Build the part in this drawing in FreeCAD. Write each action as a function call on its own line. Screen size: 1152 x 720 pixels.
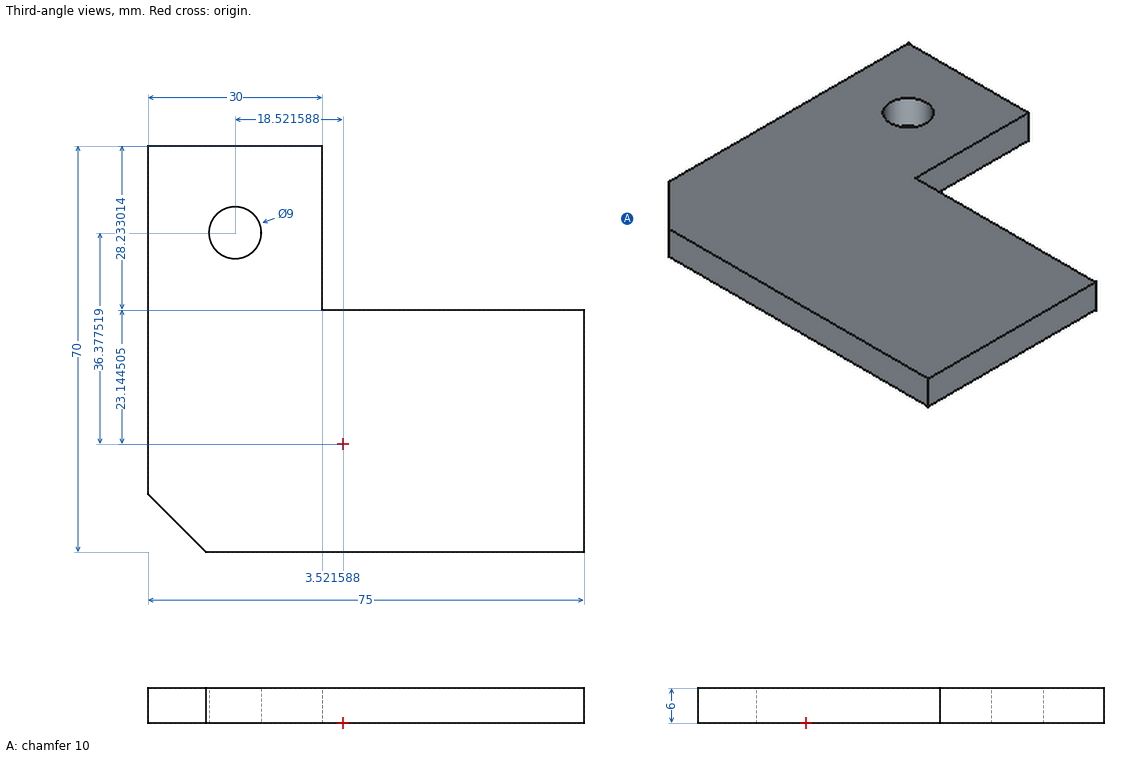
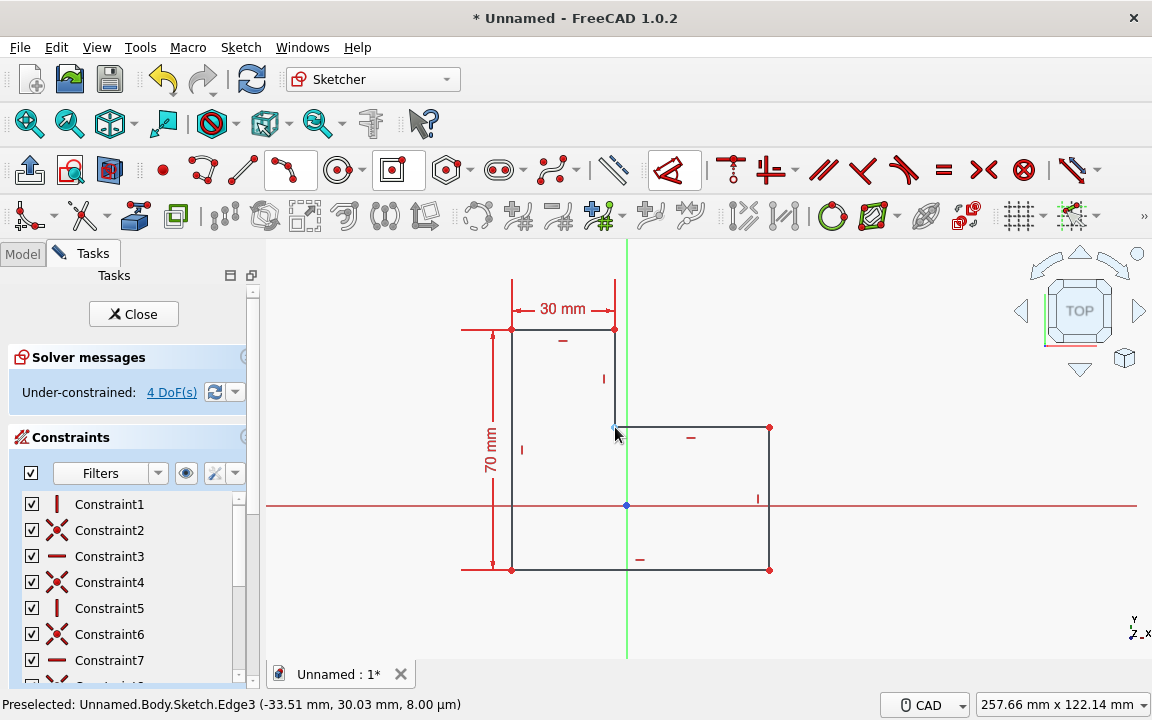
click(589, 570)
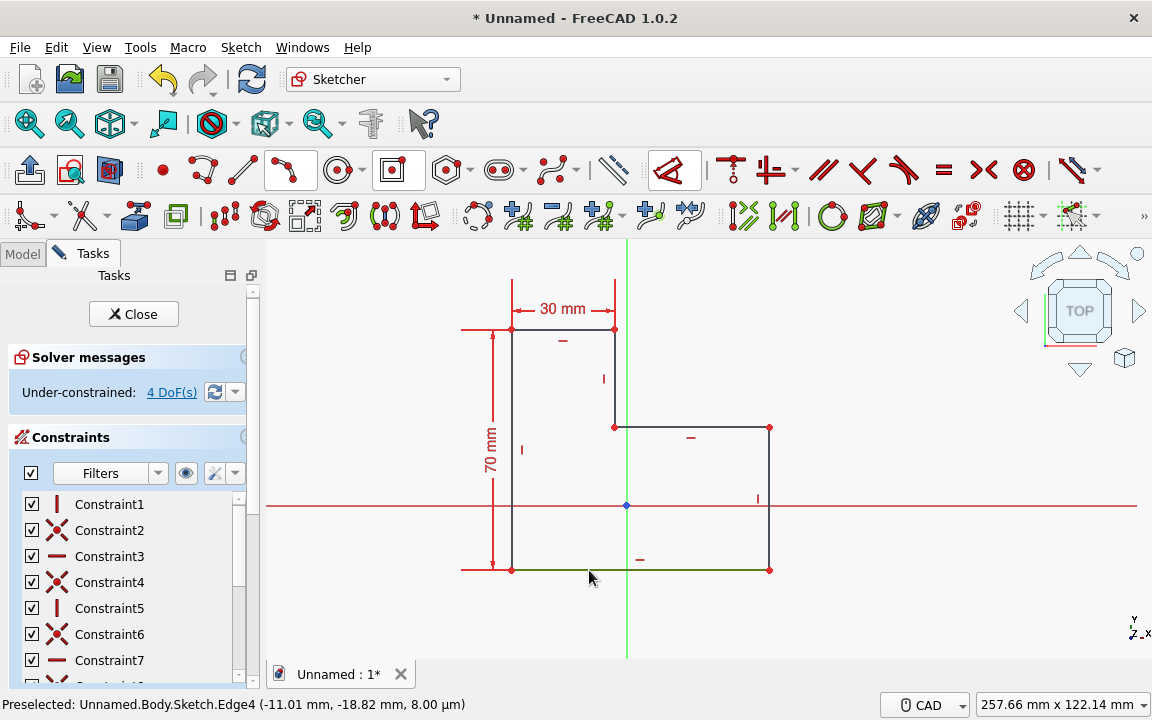
key(l)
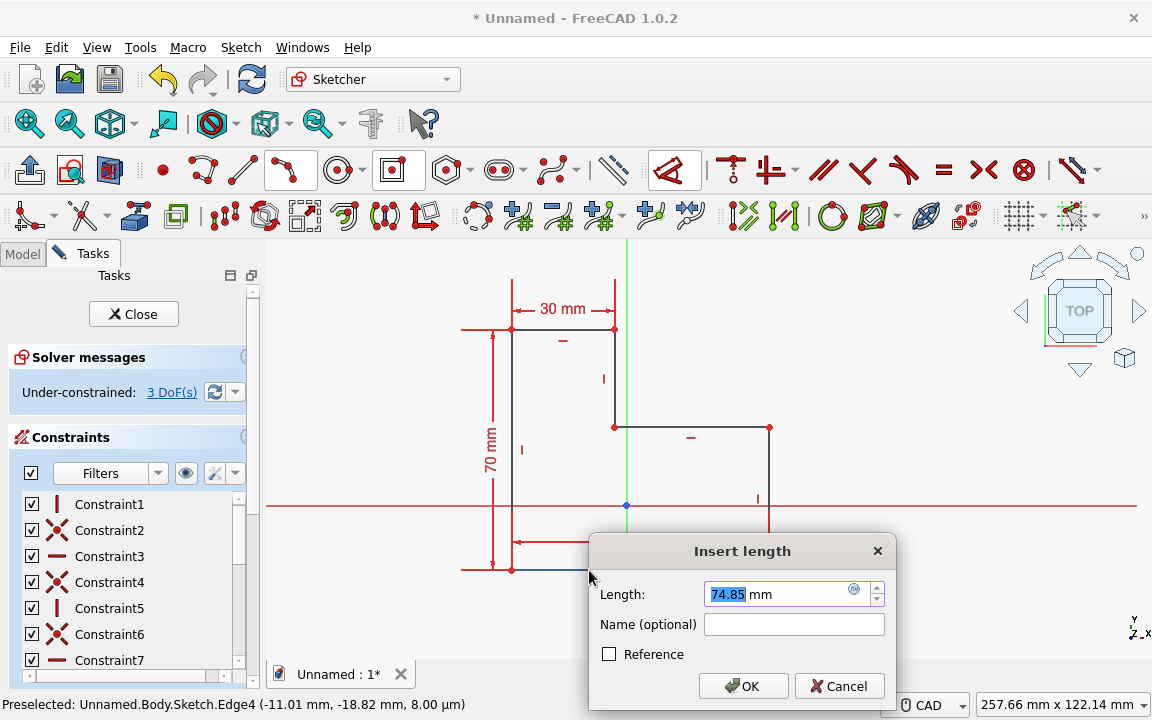
text(75)
key(Return)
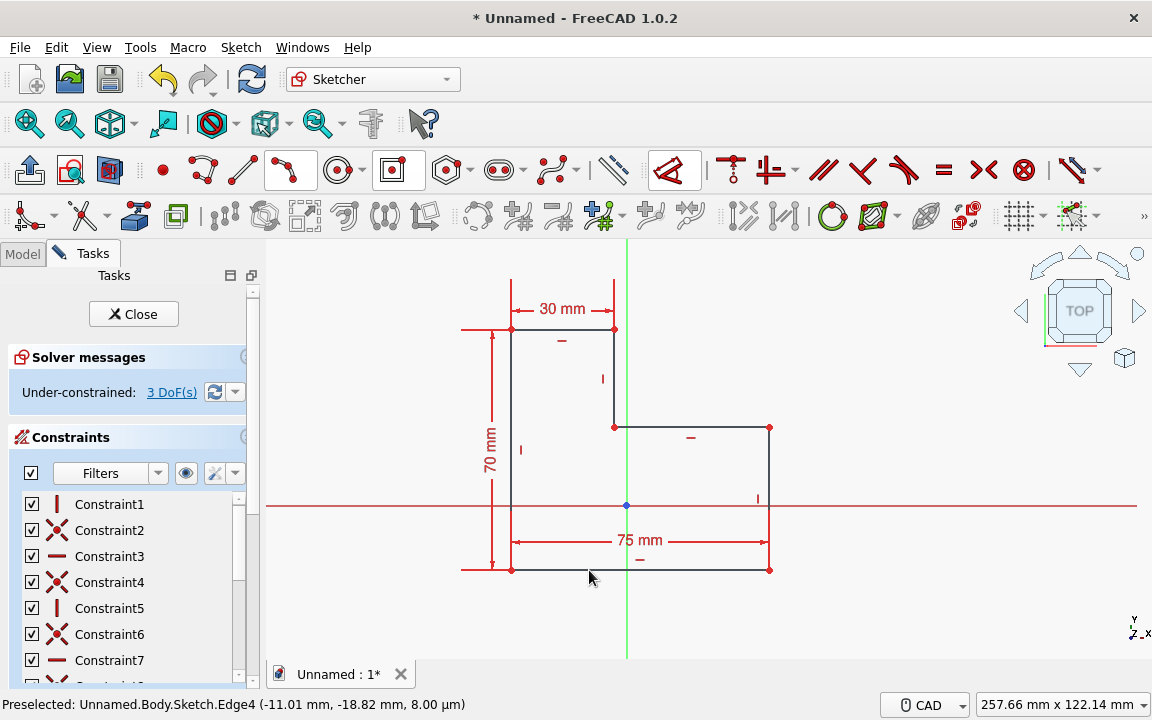
click(614, 398)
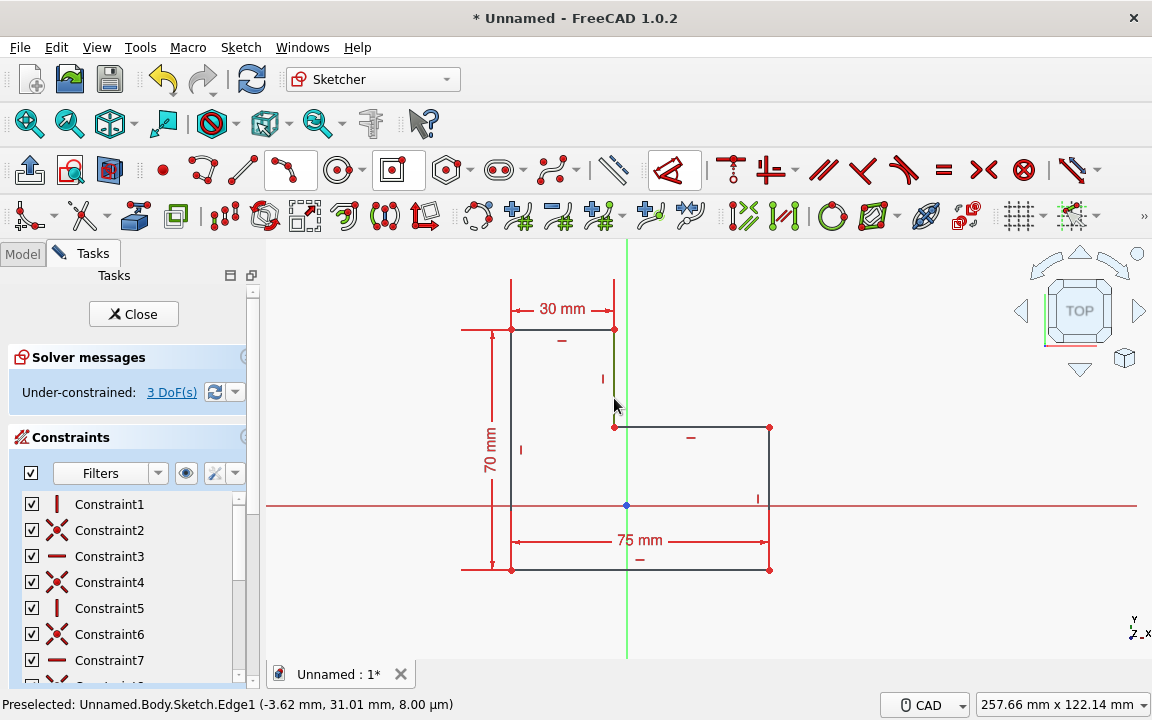
click(696, 170)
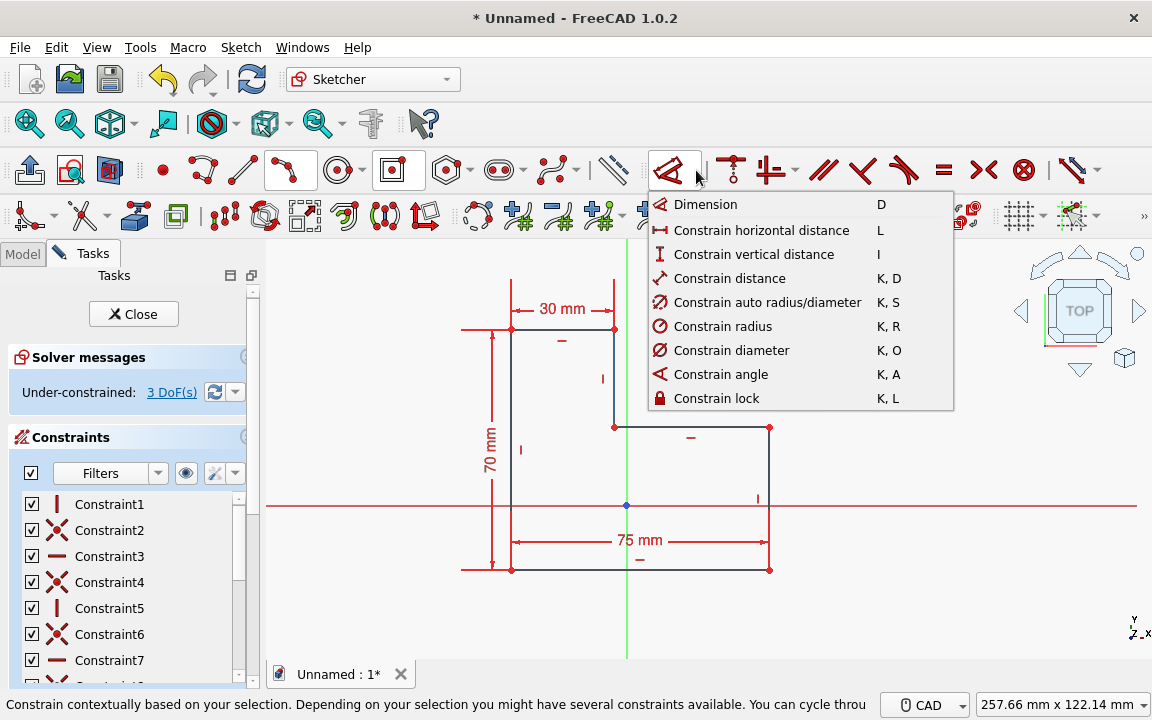
click(801, 254)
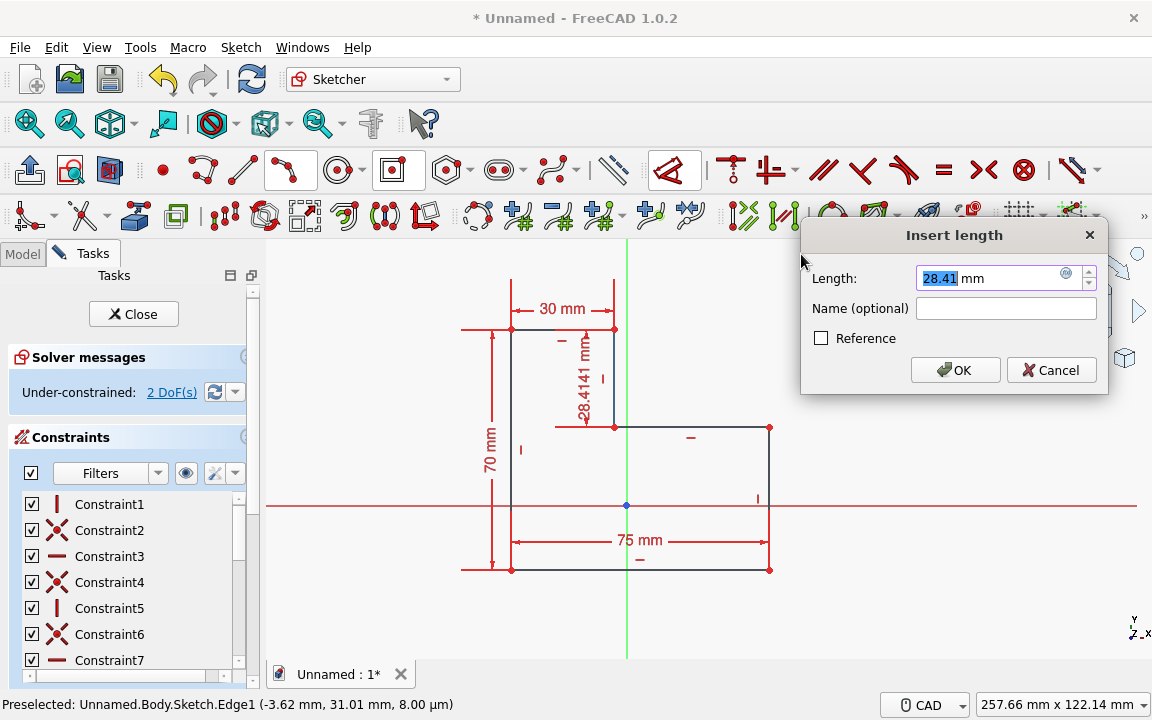
text(28.233014)
key(Return)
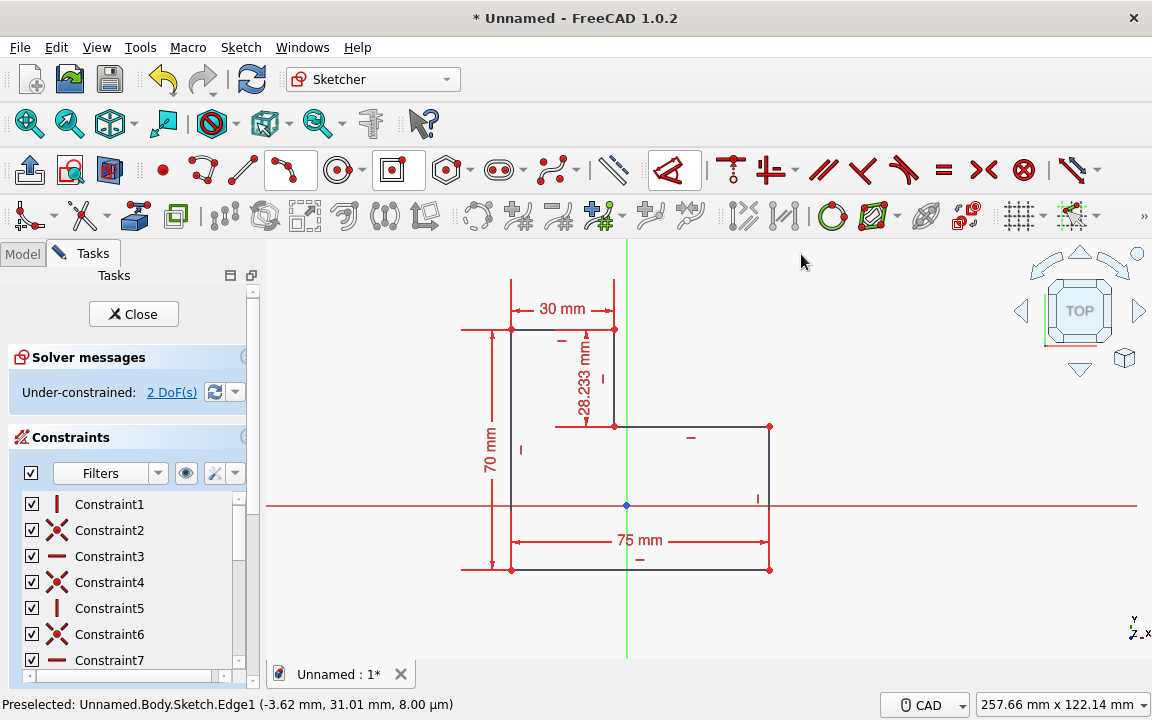
scroll(614, 427, up, 6)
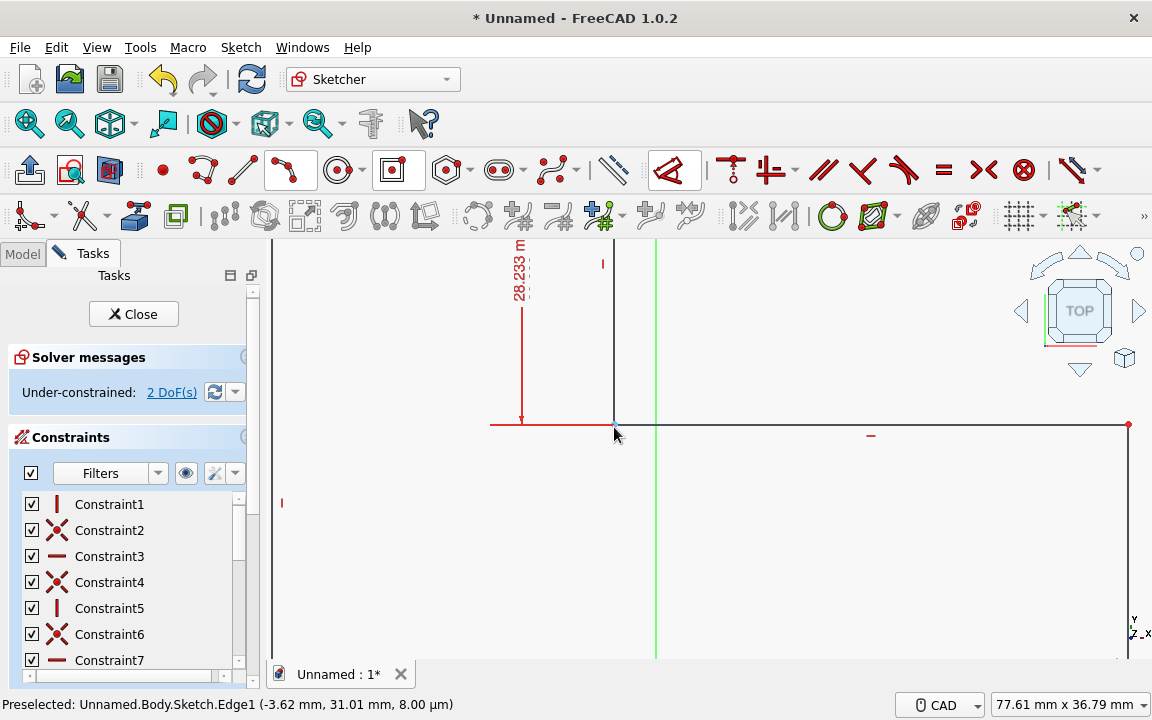
click(614, 425)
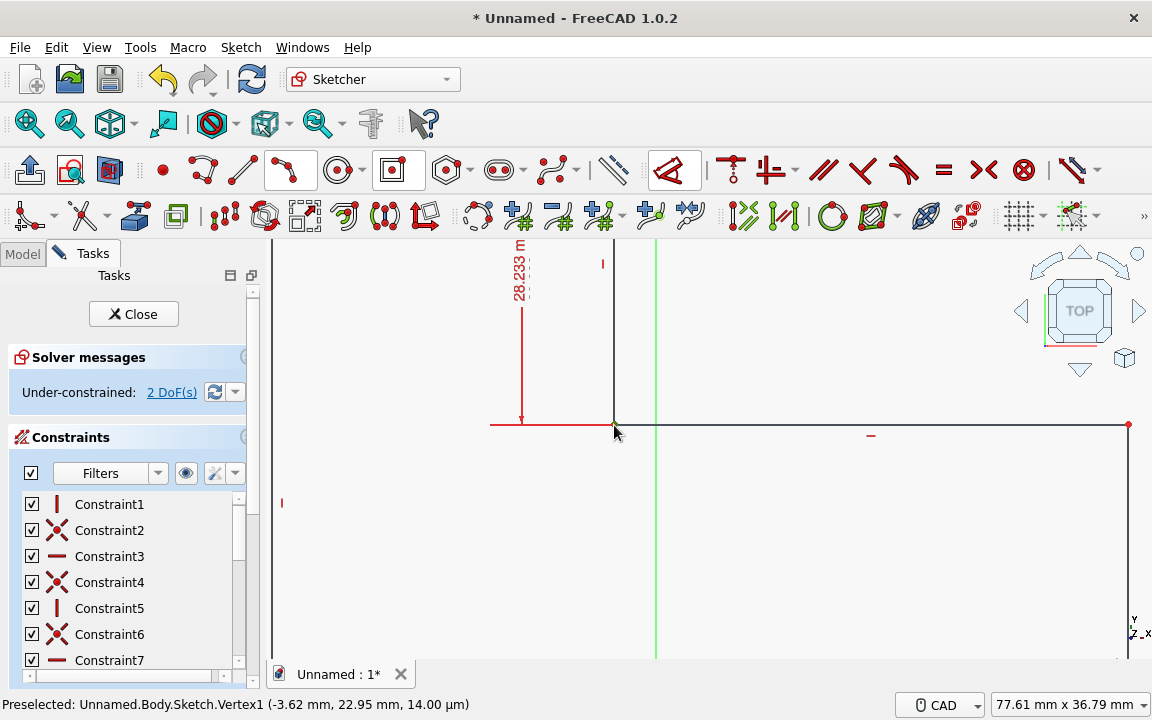
click(696, 170)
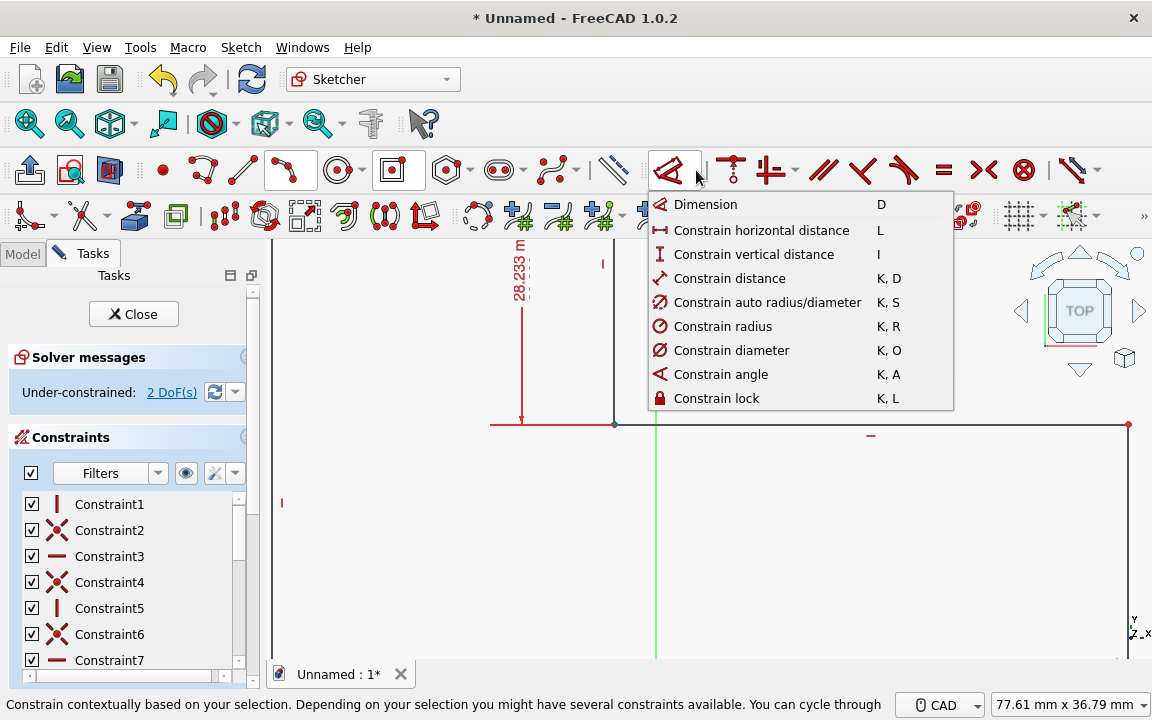
click(801, 230)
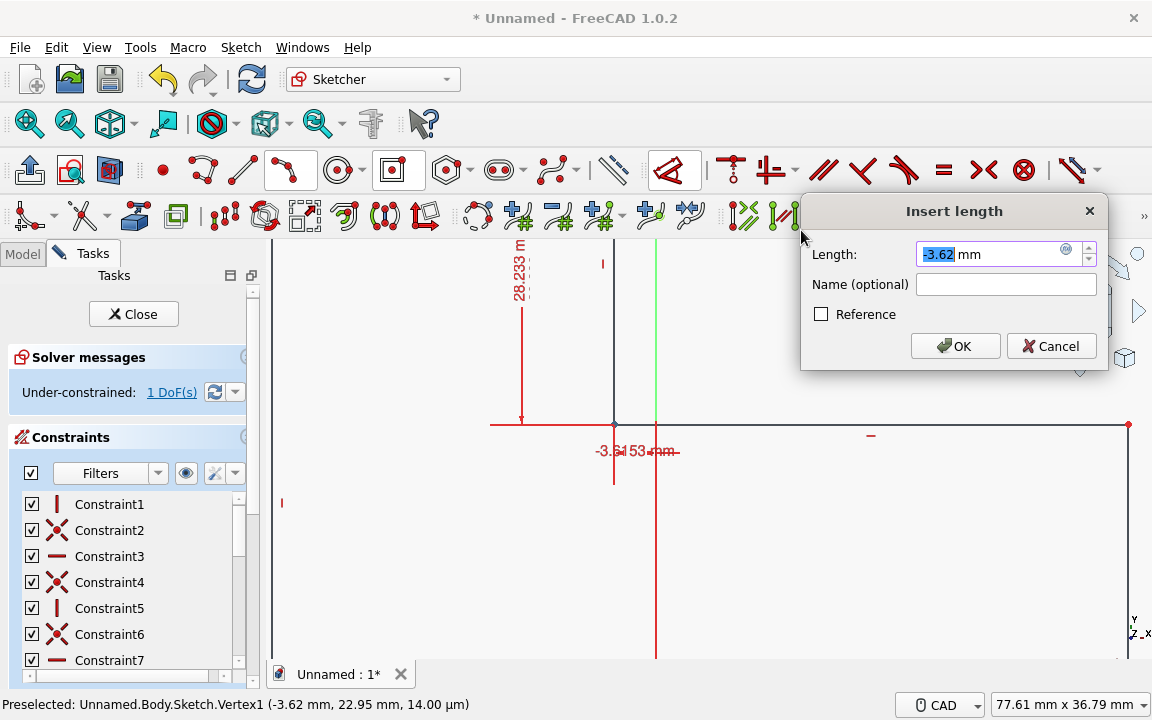
text(-3.521588)
key(Return)